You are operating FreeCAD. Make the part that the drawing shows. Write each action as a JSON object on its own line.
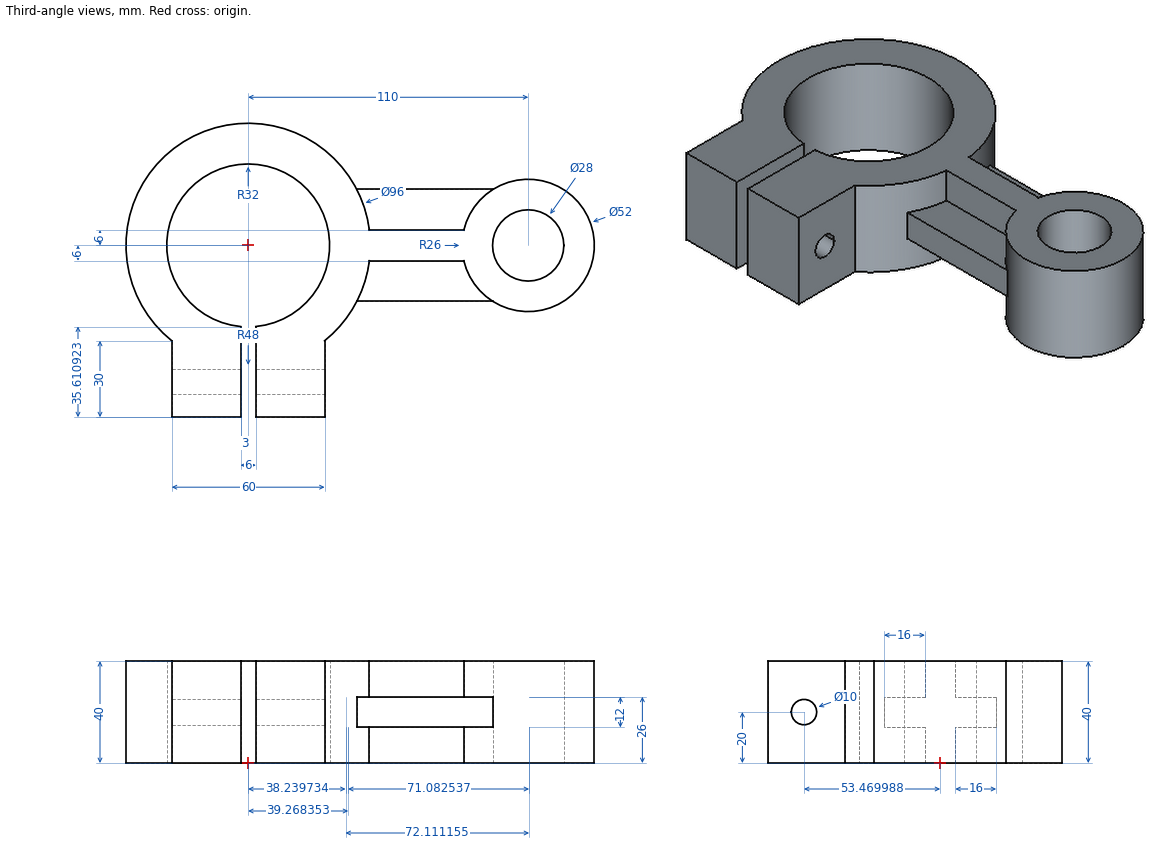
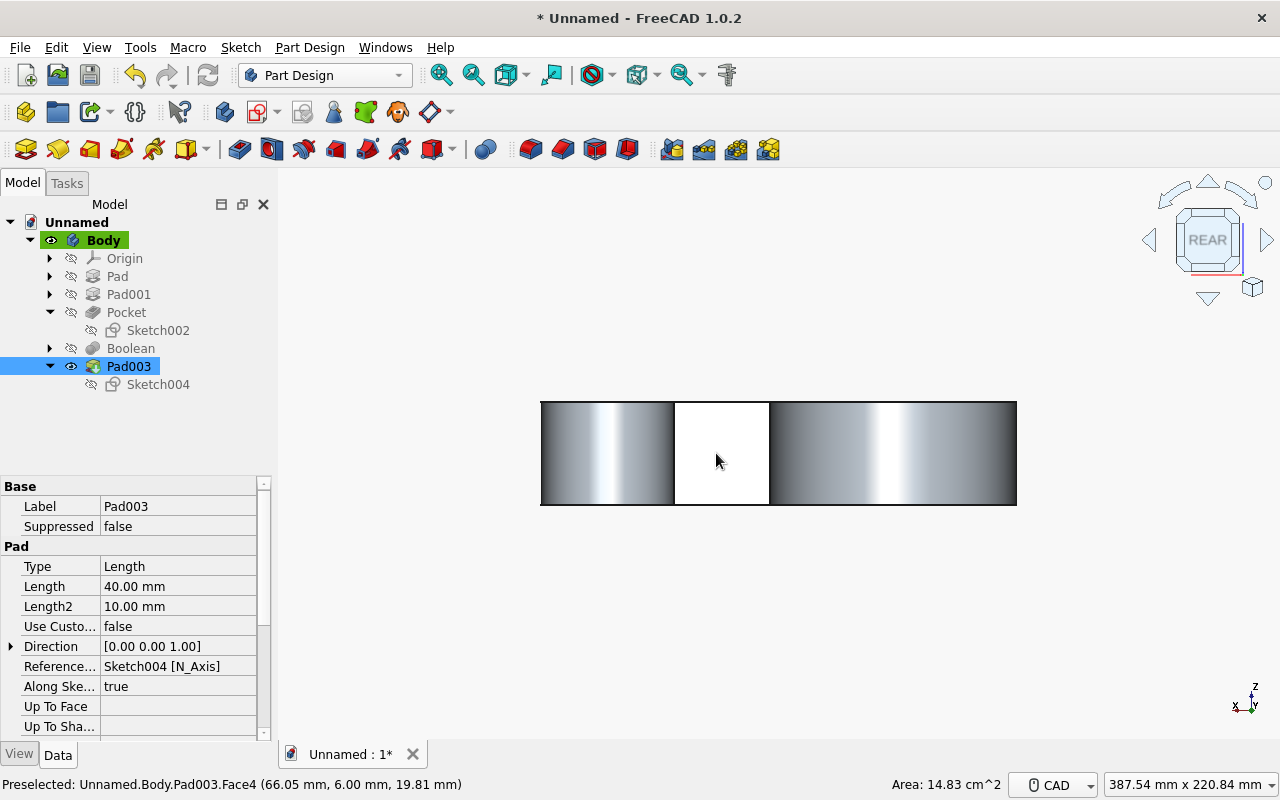
{"action": "left_click", "coordinate": [258, 112]}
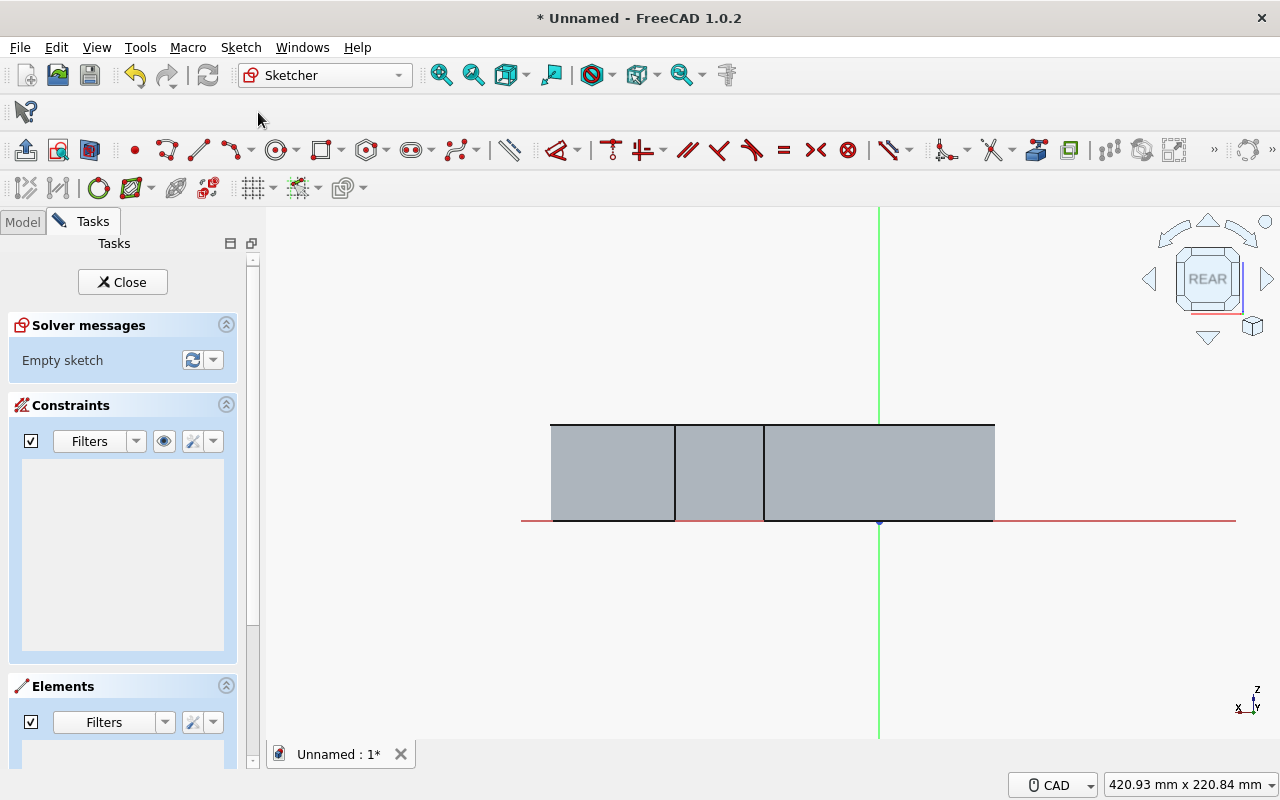
{"action": "left_click", "coordinate": [90, 150]}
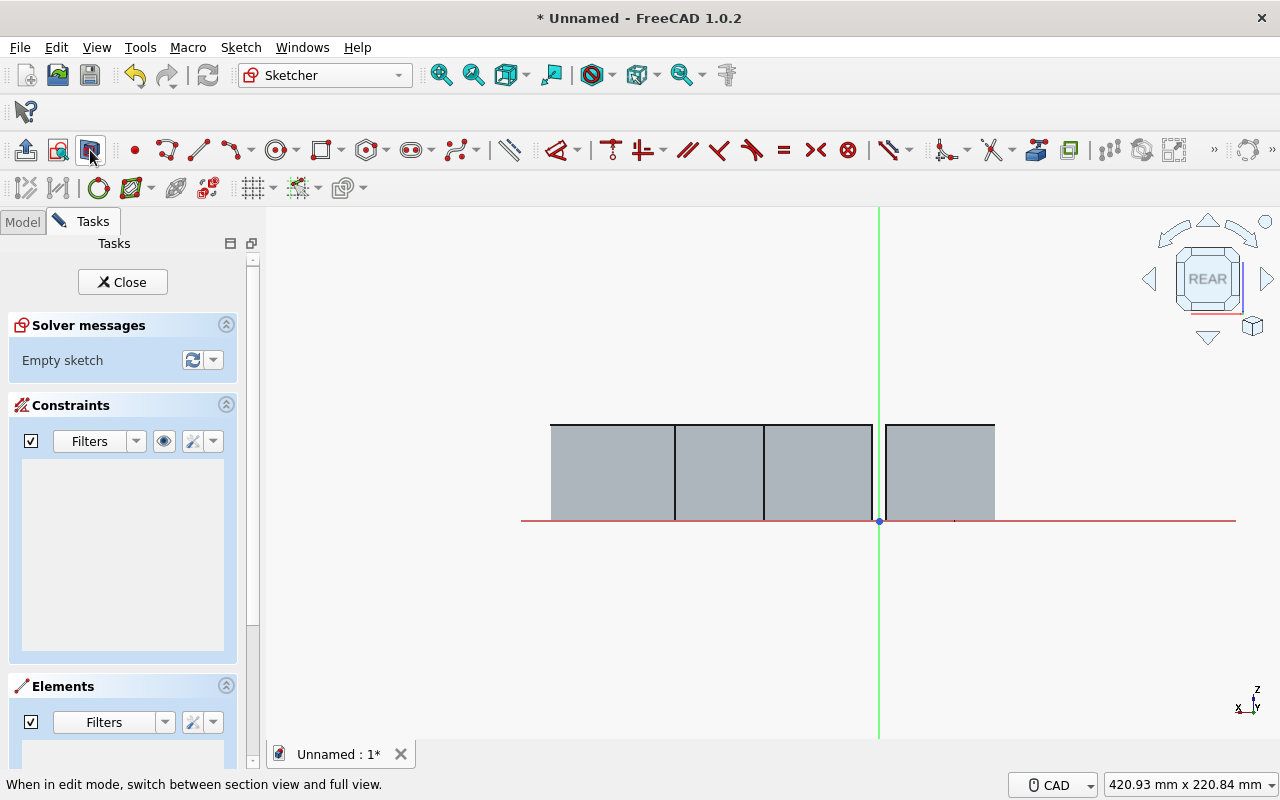
{"action": "scroll", "coordinate": [780, 504], "scroll_direction": "up", "scroll_amount": 4}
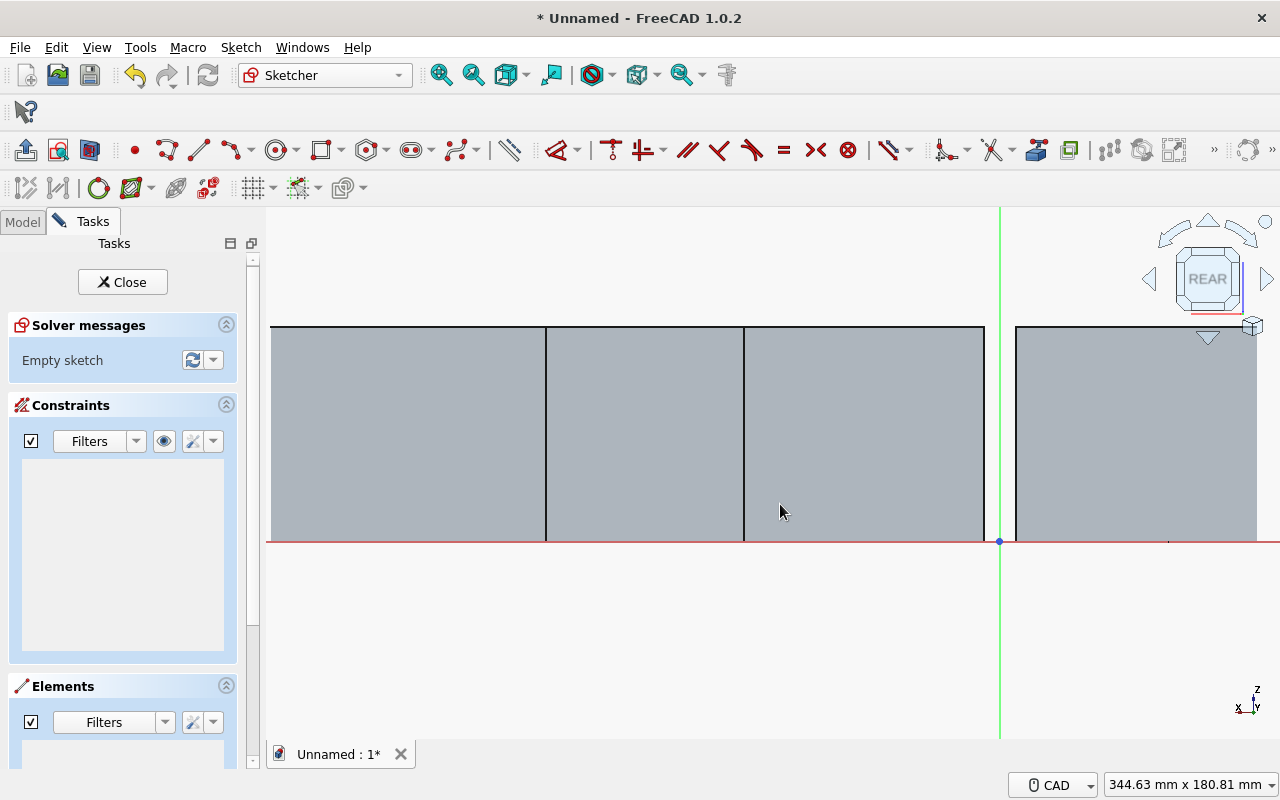
{"action": "left_click", "coordinate": [322, 150]}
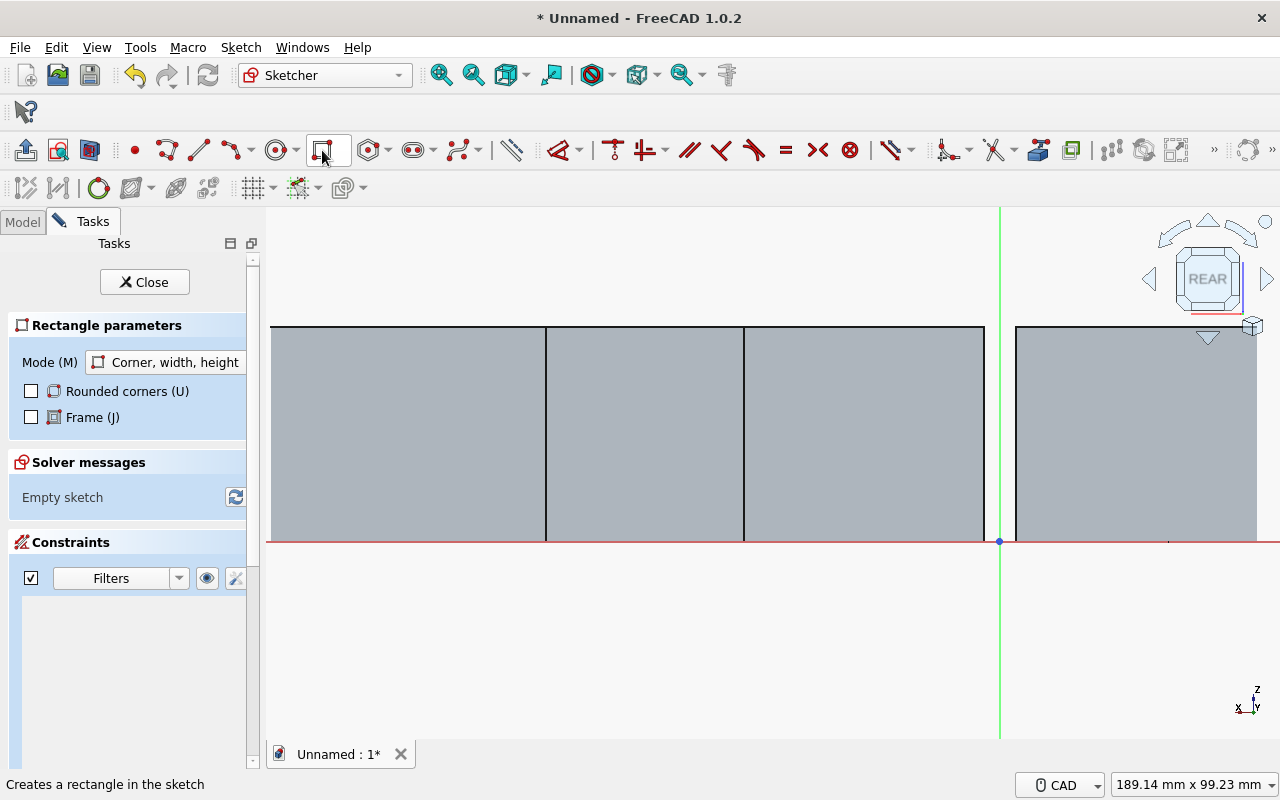
{"action": "left_click", "coordinate": [408, 402]}
{"action": "left_click", "coordinate": [789, 466]}
{"action": "key", "text": "Escape"}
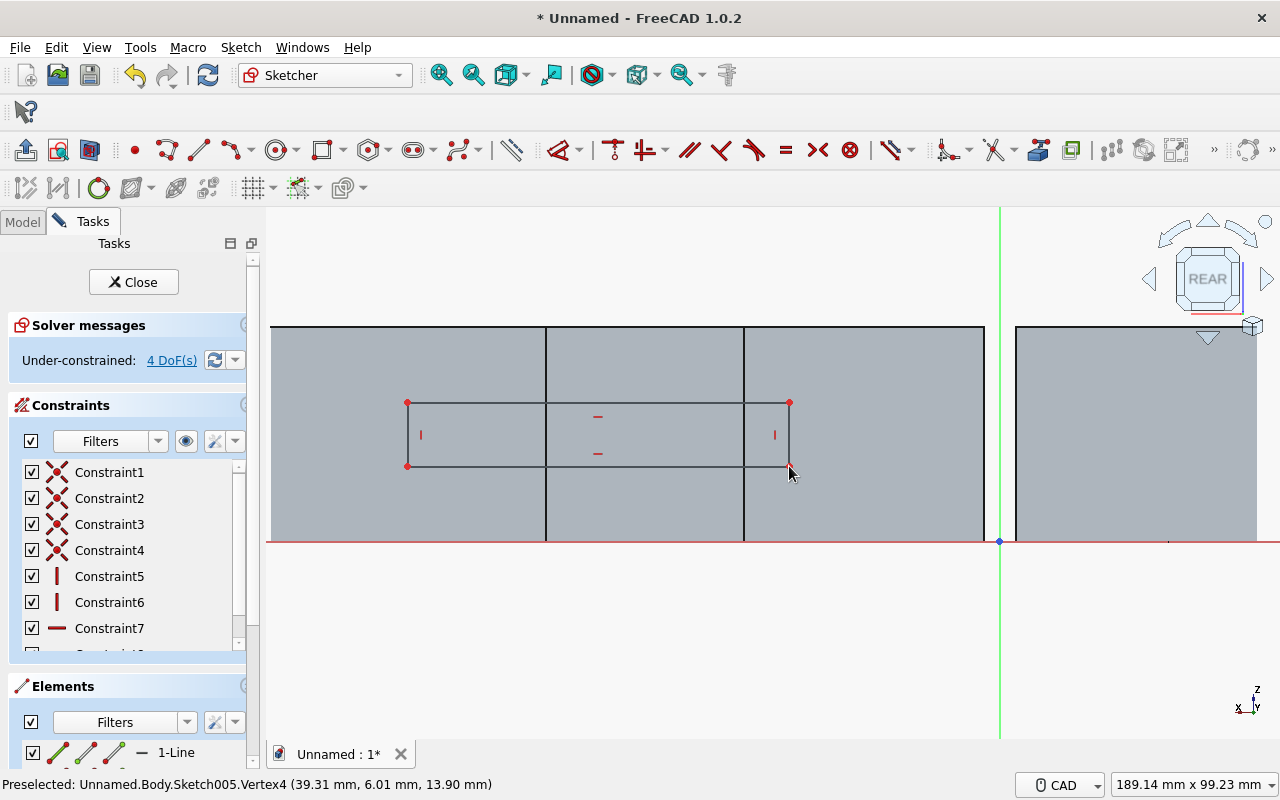
{"action": "left_click", "coordinate": [558, 150]}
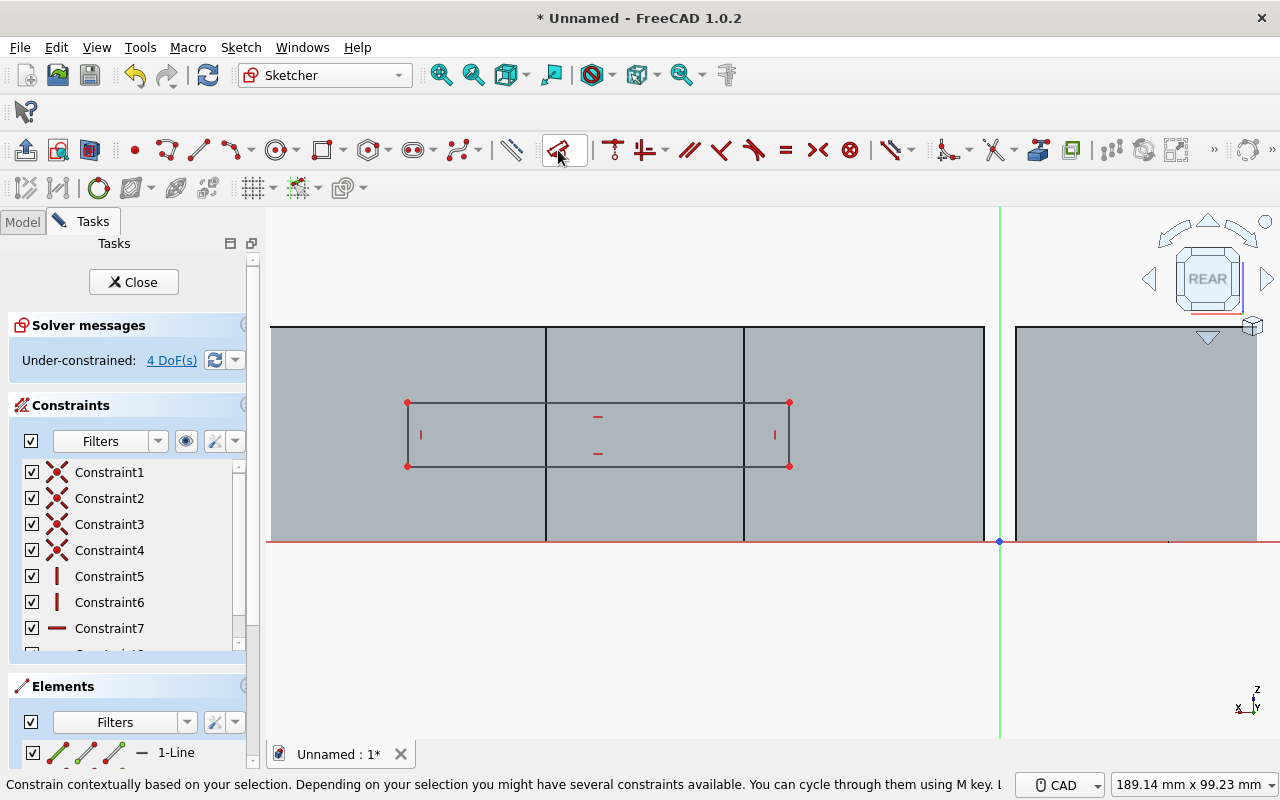
{"action": "left_click", "coordinate": [408, 422]}
{"action": "left_click", "coordinate": [374, 435]}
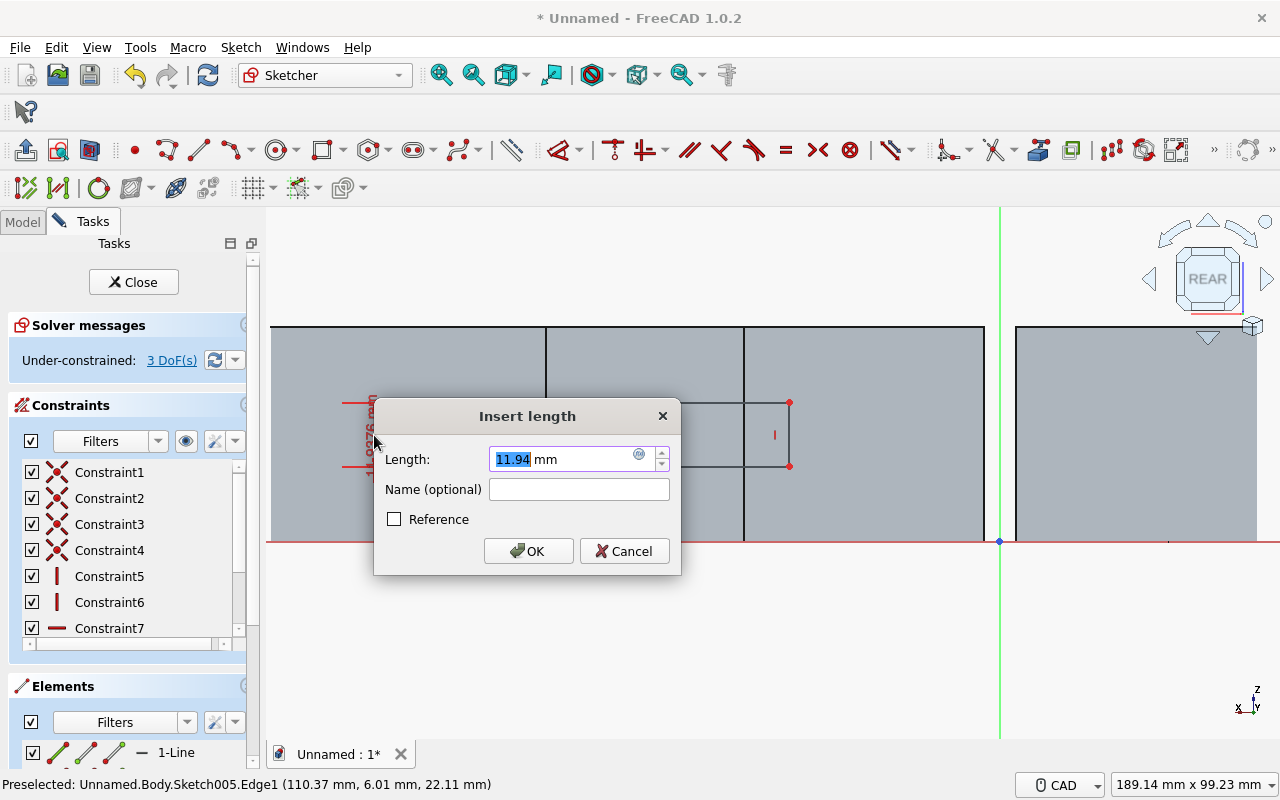
{"action": "type", "text": "12"}
{"action": "key", "text": "Return"}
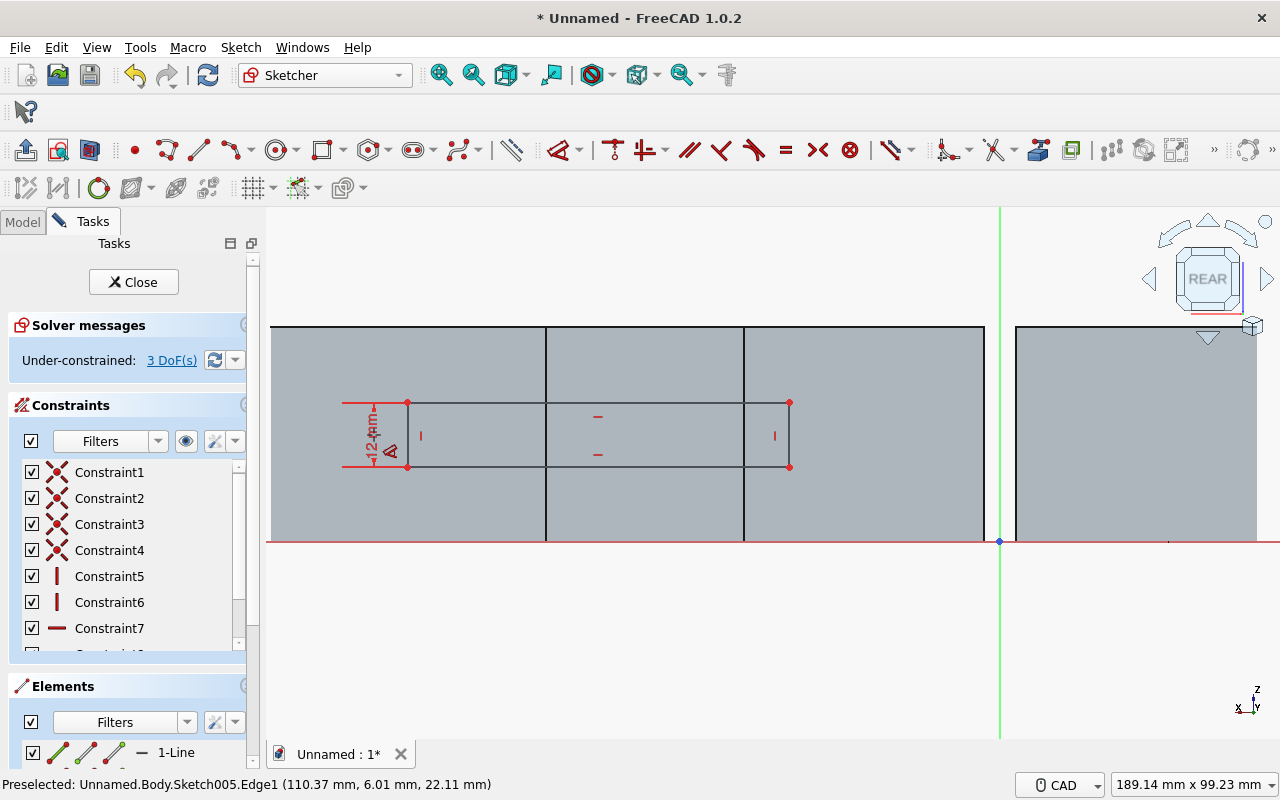
{"action": "left_click", "coordinate": [408, 403]}
{"action": "left_click", "coordinate": [374, 472]}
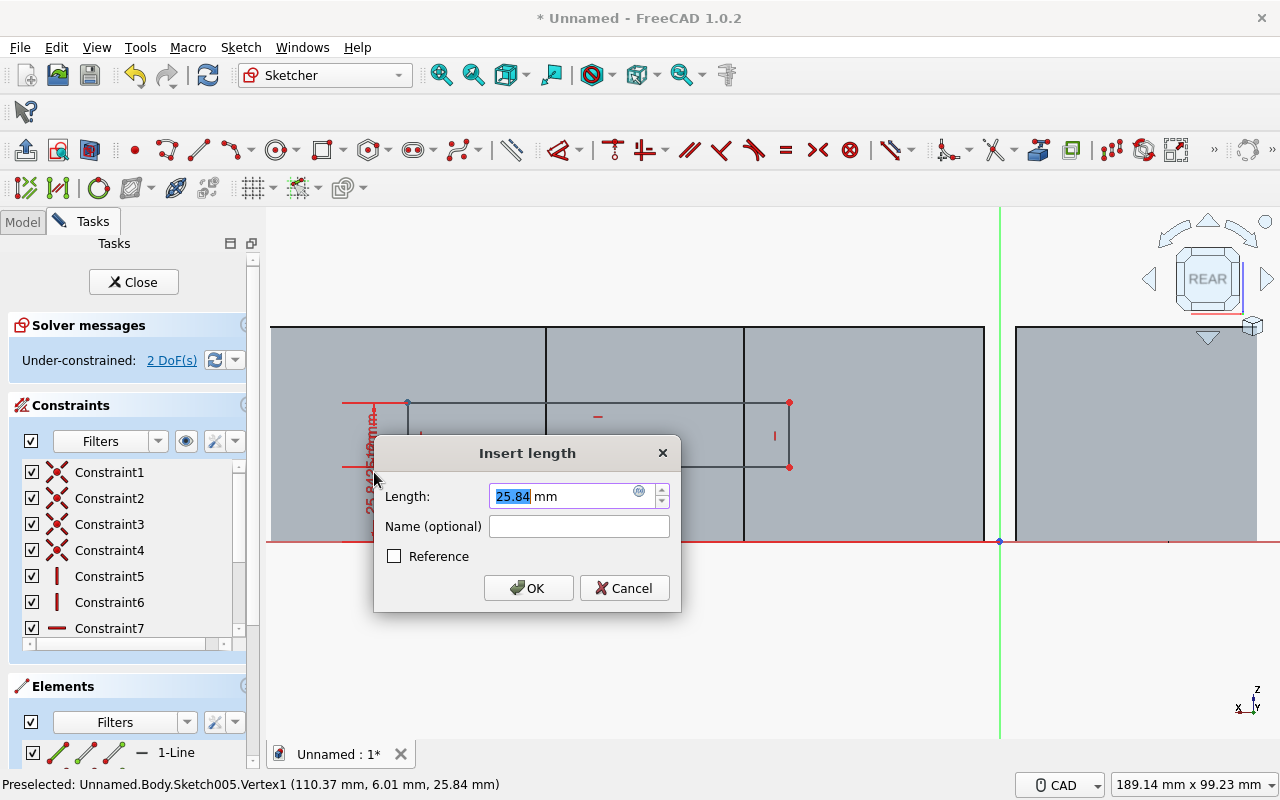
{"action": "type", "text": "26"}
{"action": "key", "text": "Return"}